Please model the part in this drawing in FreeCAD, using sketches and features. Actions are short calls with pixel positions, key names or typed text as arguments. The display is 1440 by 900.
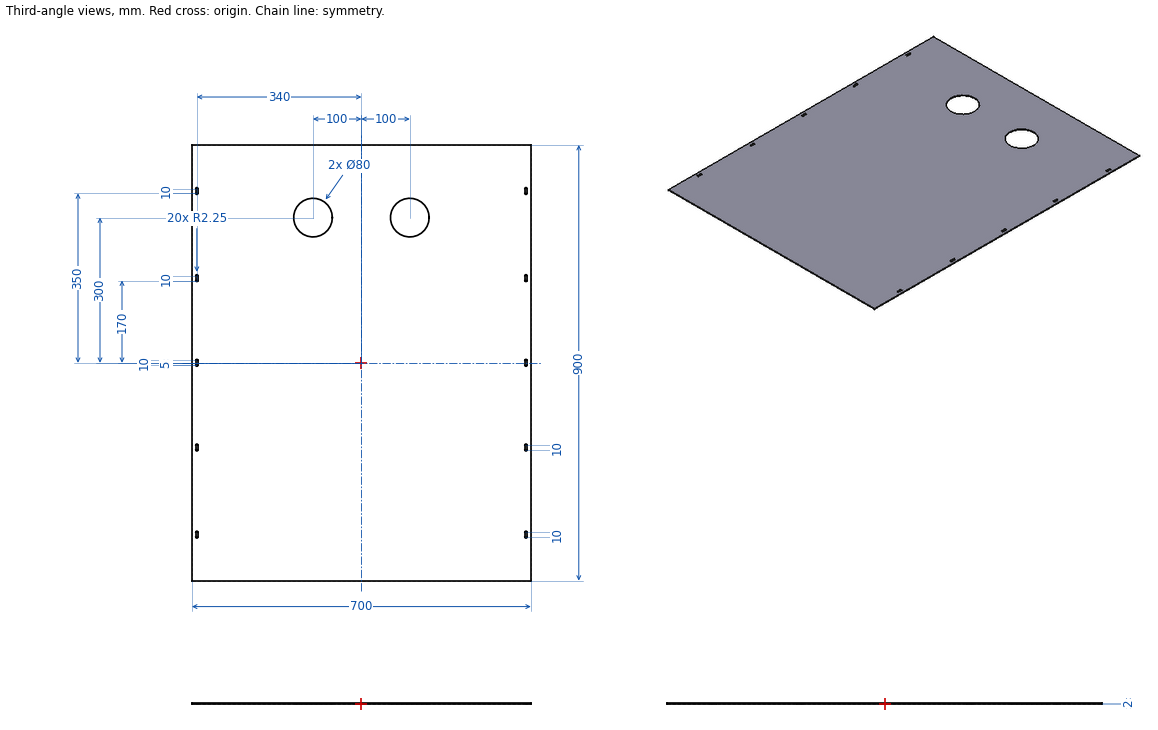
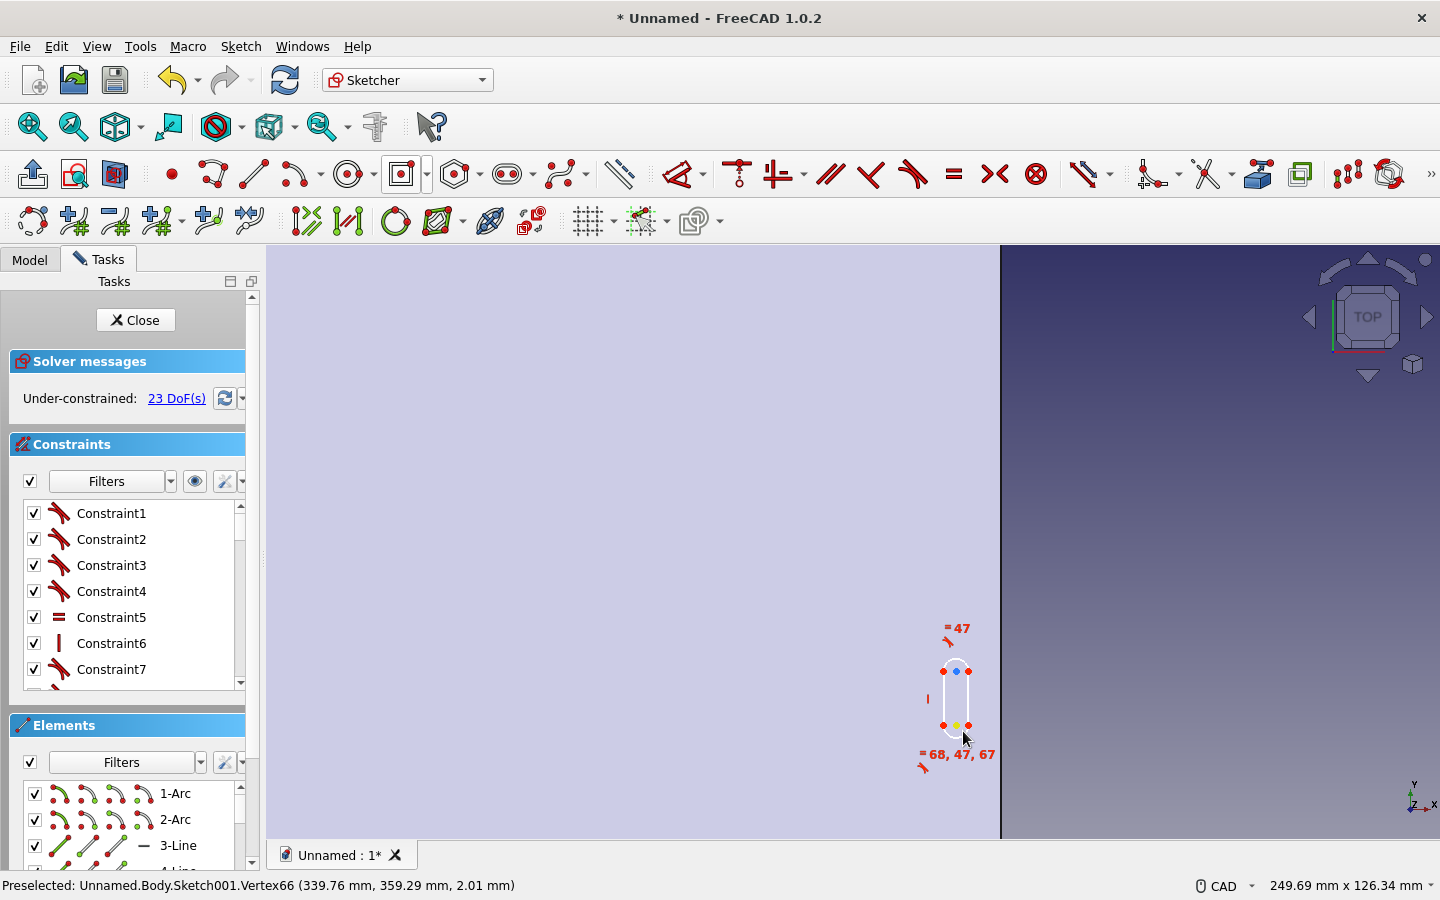
click(956, 726)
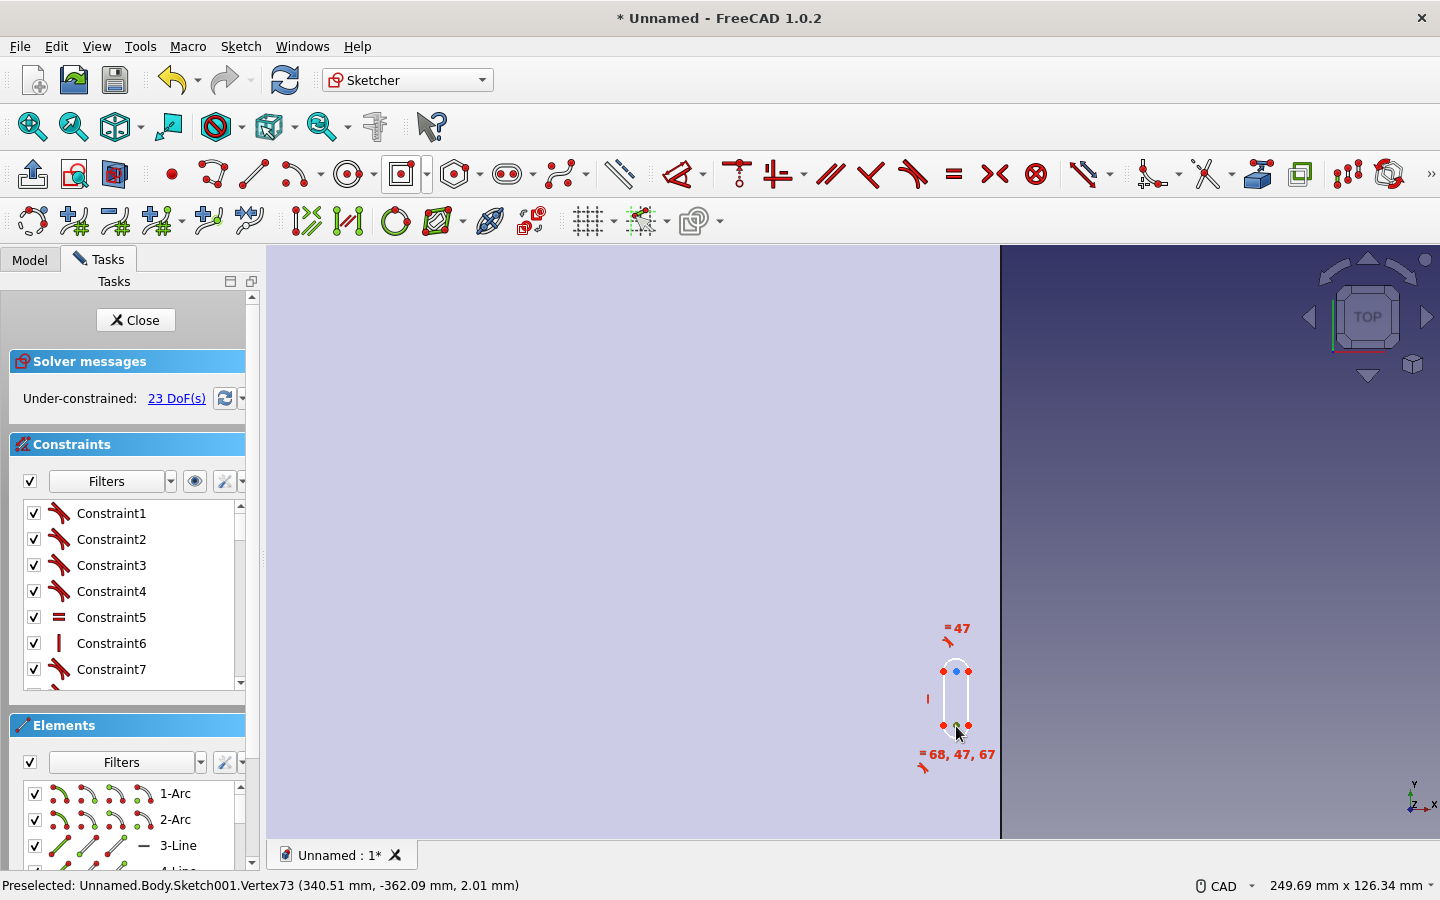
scroll(963, 731, down, 11)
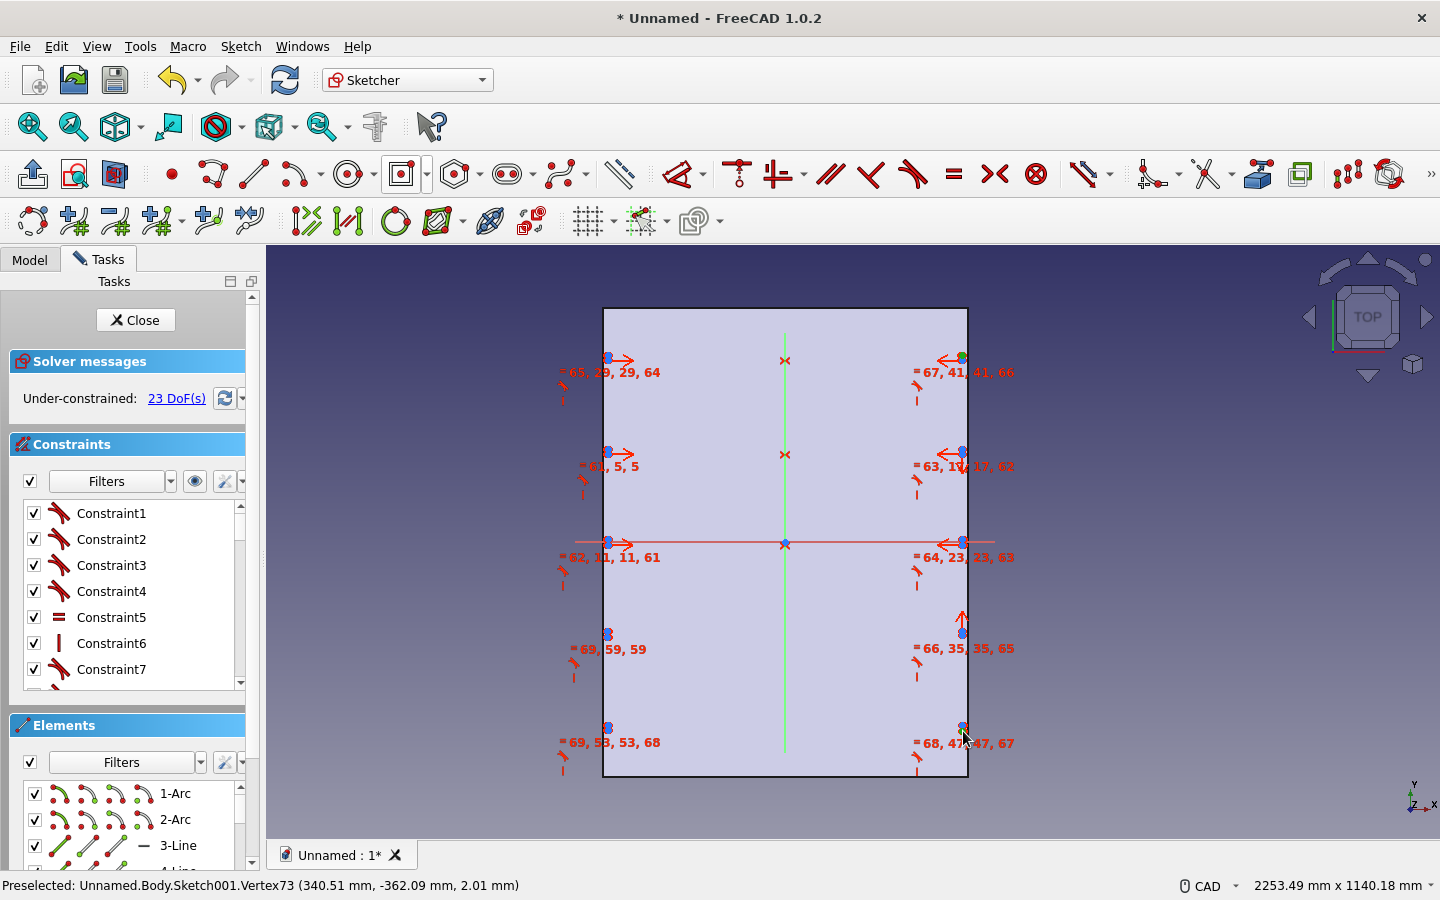
click(574, 542)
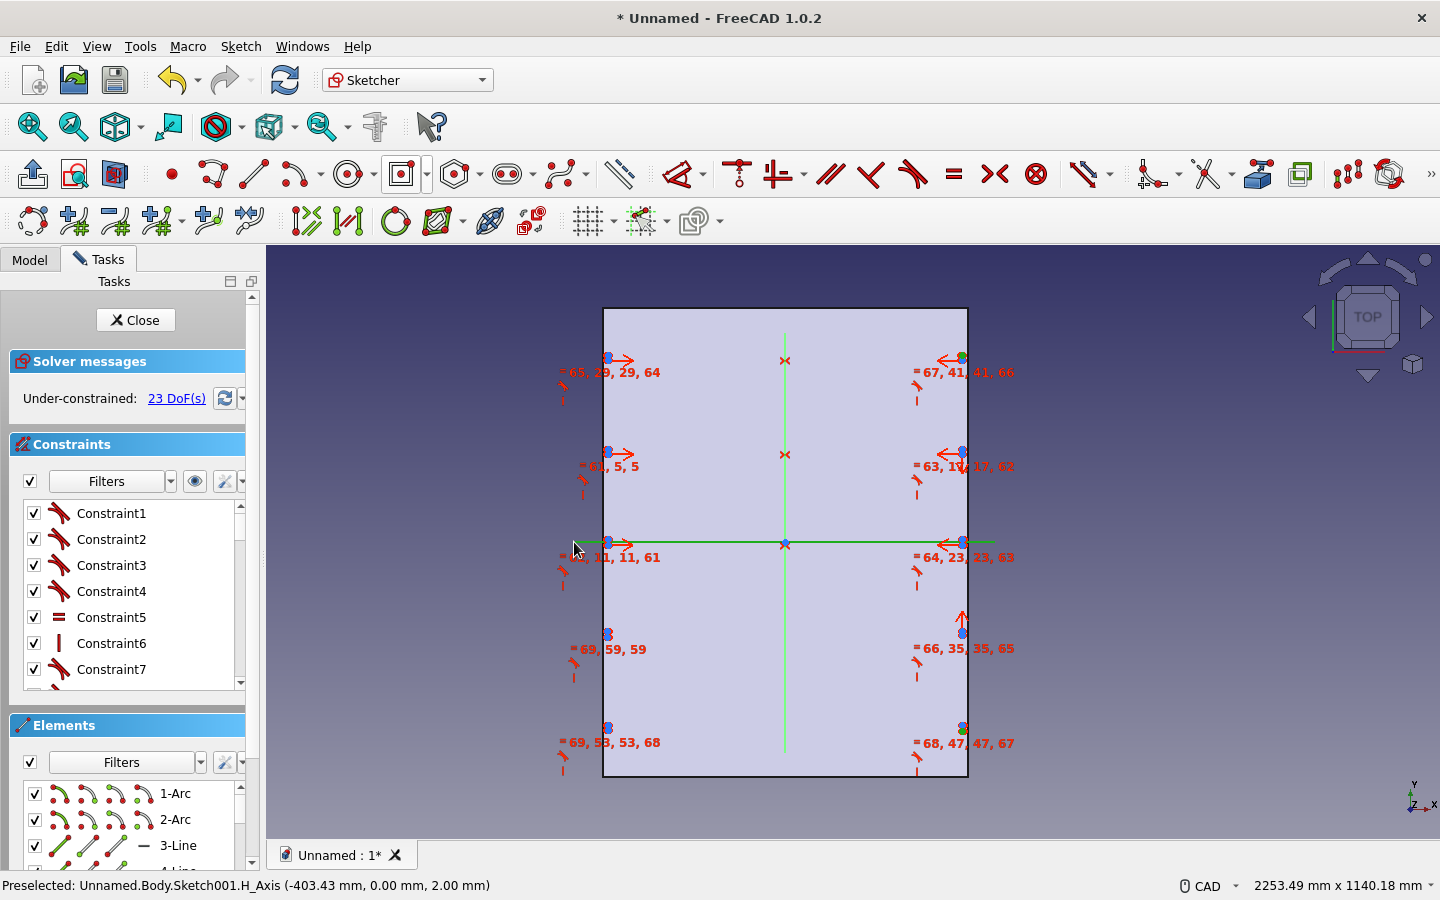
key(s)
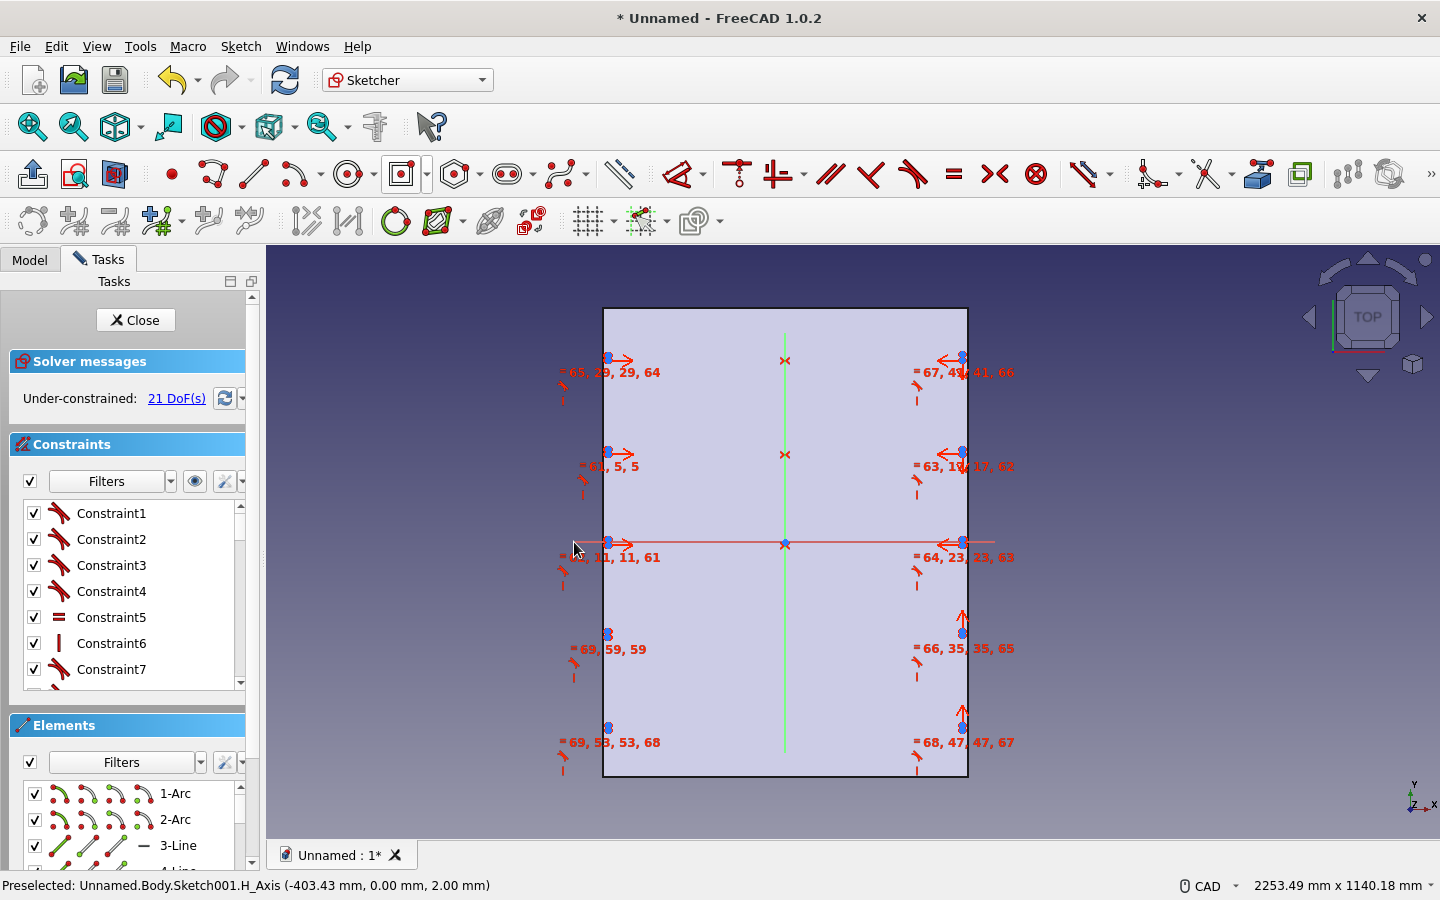
scroll(608, 355, up, 11)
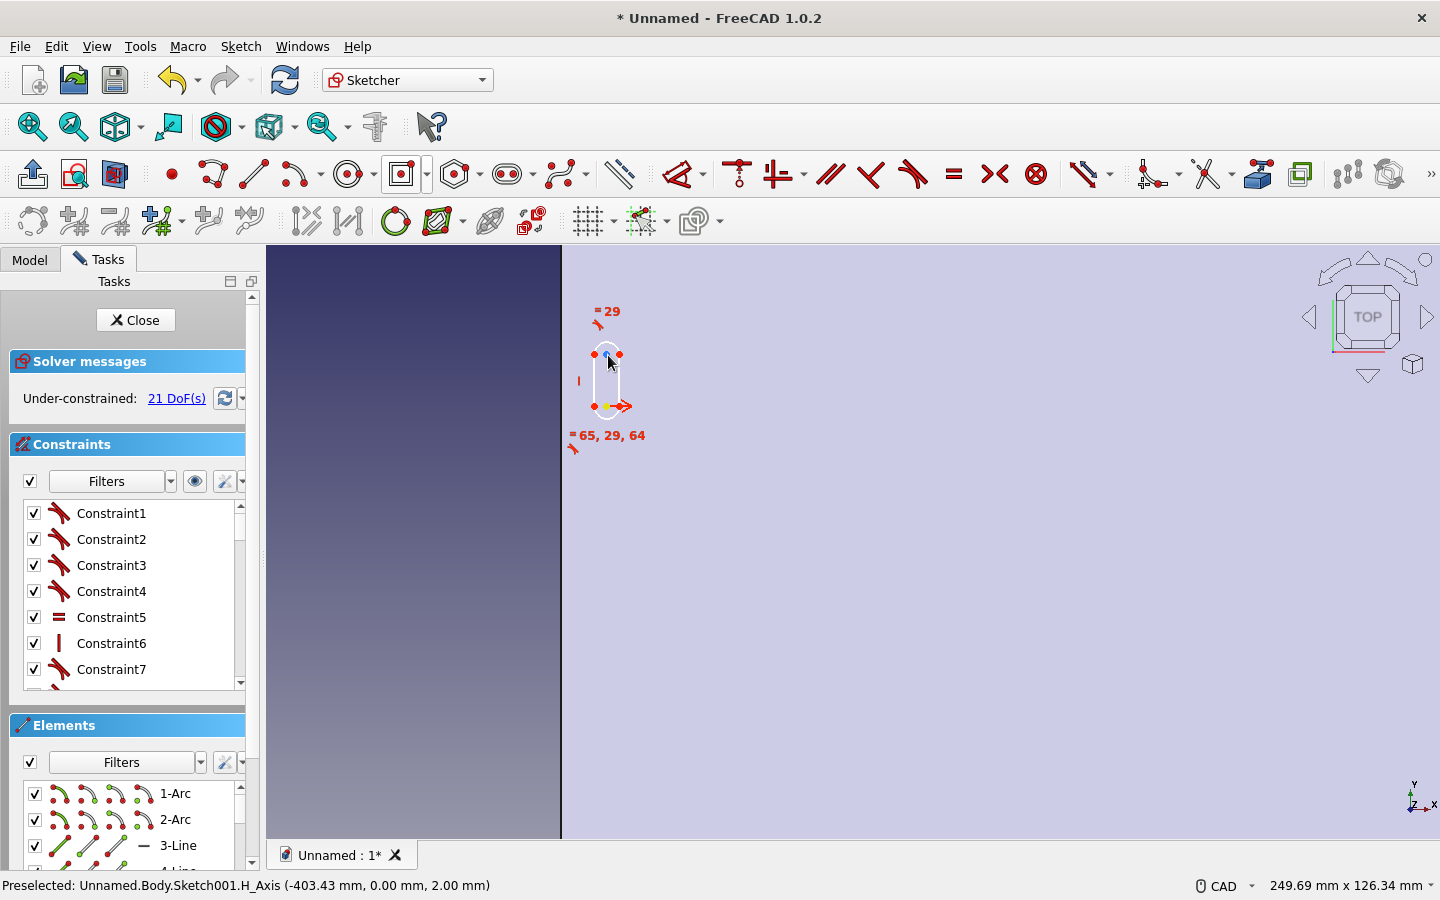
click(607, 355)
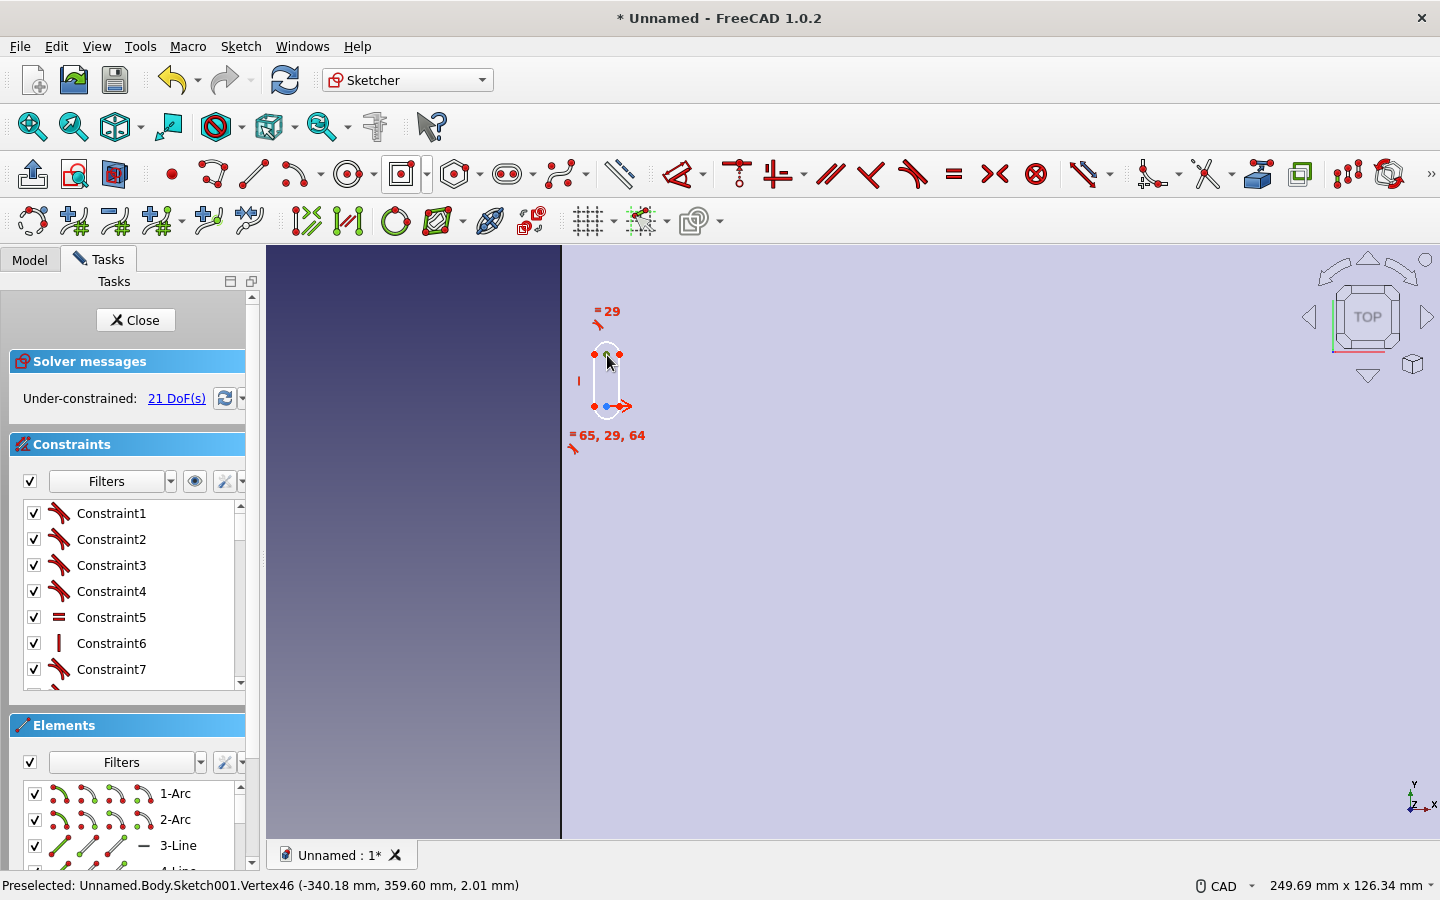
scroll(607, 355, down, 11)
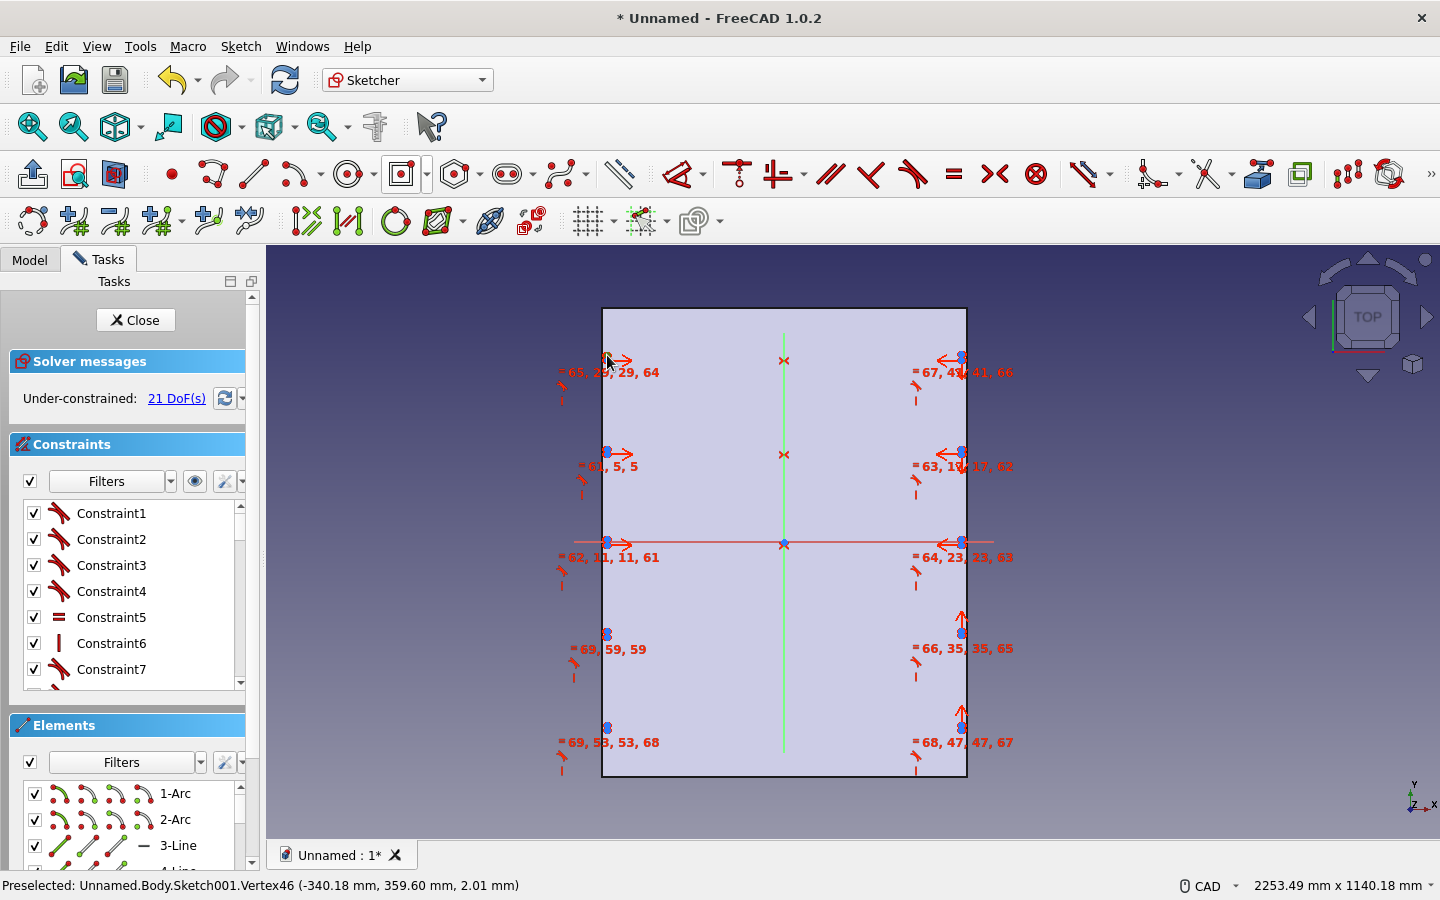
scroll(608, 731, up, 11)